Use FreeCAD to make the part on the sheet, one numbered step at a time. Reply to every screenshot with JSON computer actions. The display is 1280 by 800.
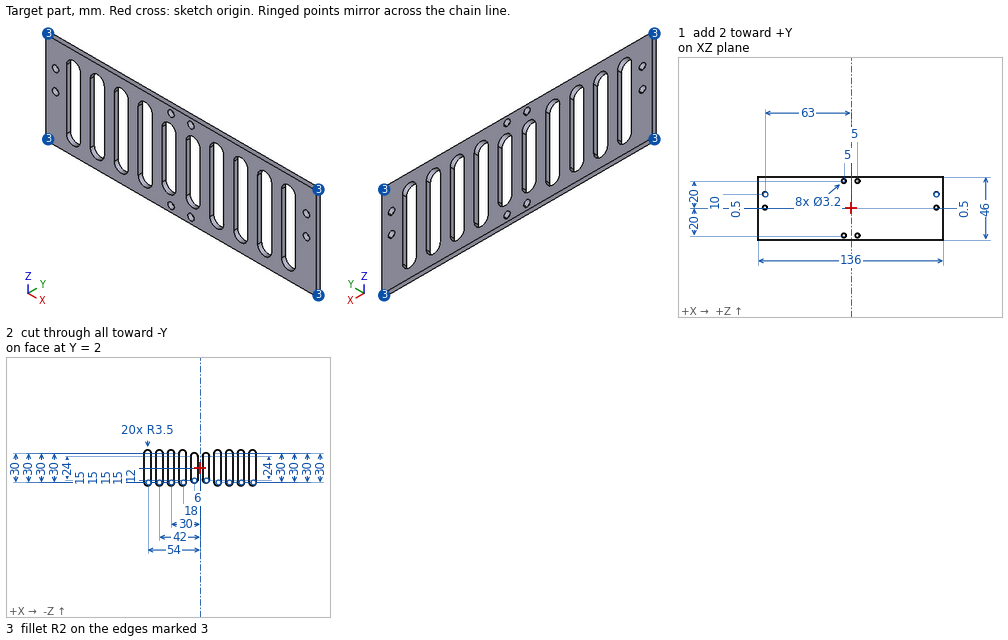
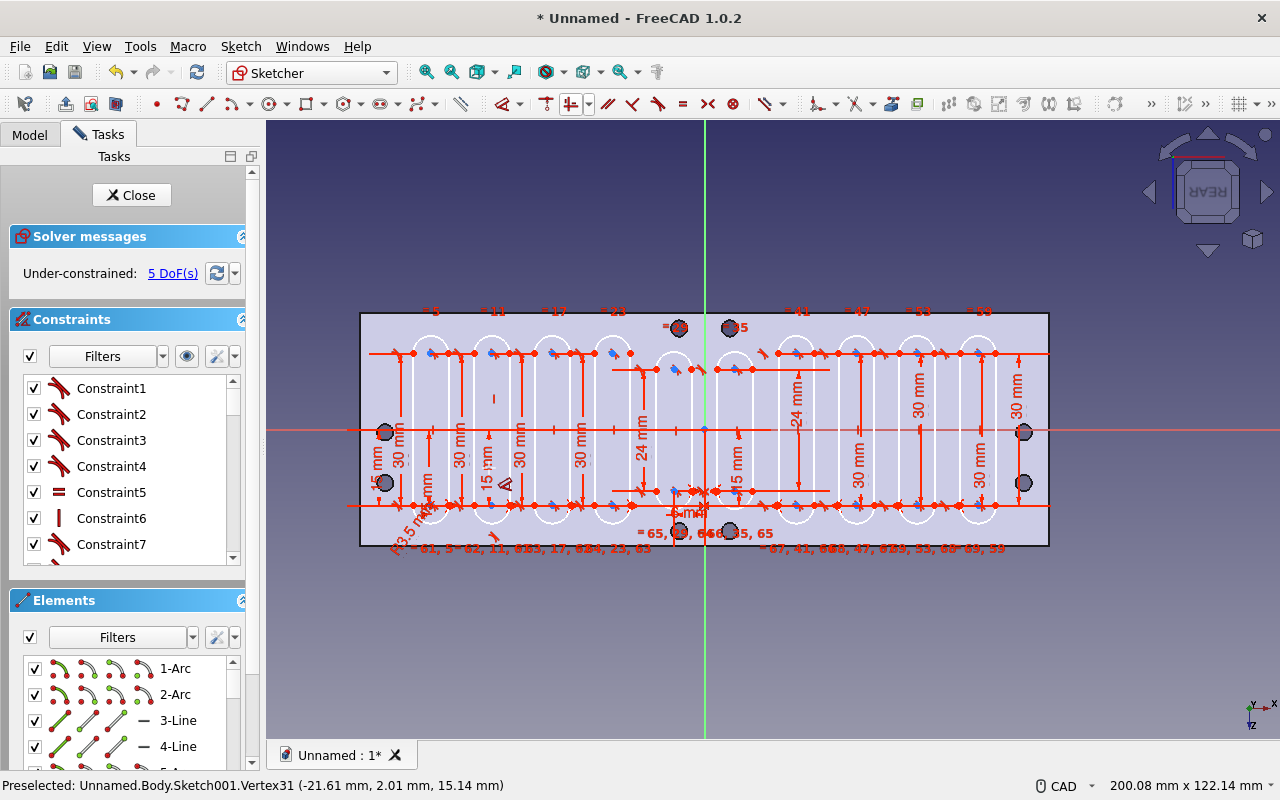
{"action": "left_click", "coordinate": [656, 491]}
{"action": "left_click", "coordinate": [739, 446]}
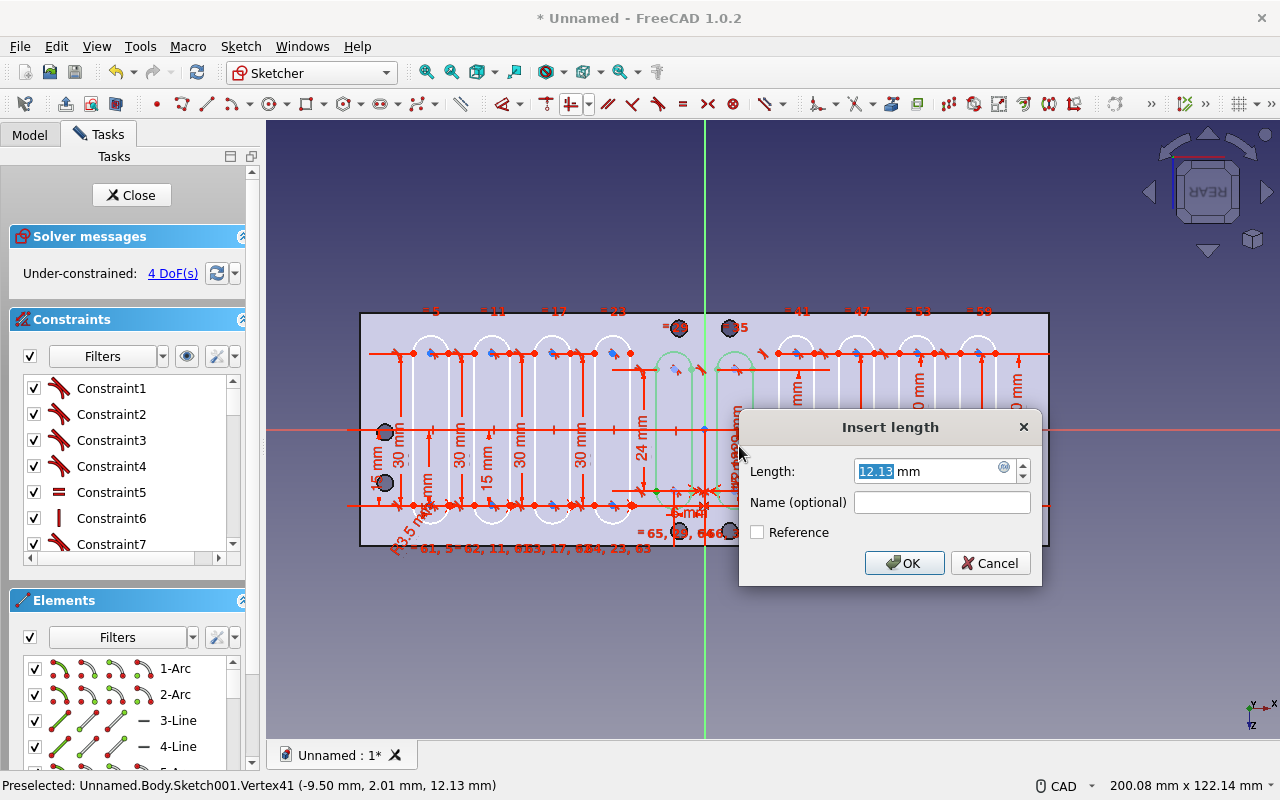
{"action": "type", "text": "12"}
{"action": "key", "text": "Return"}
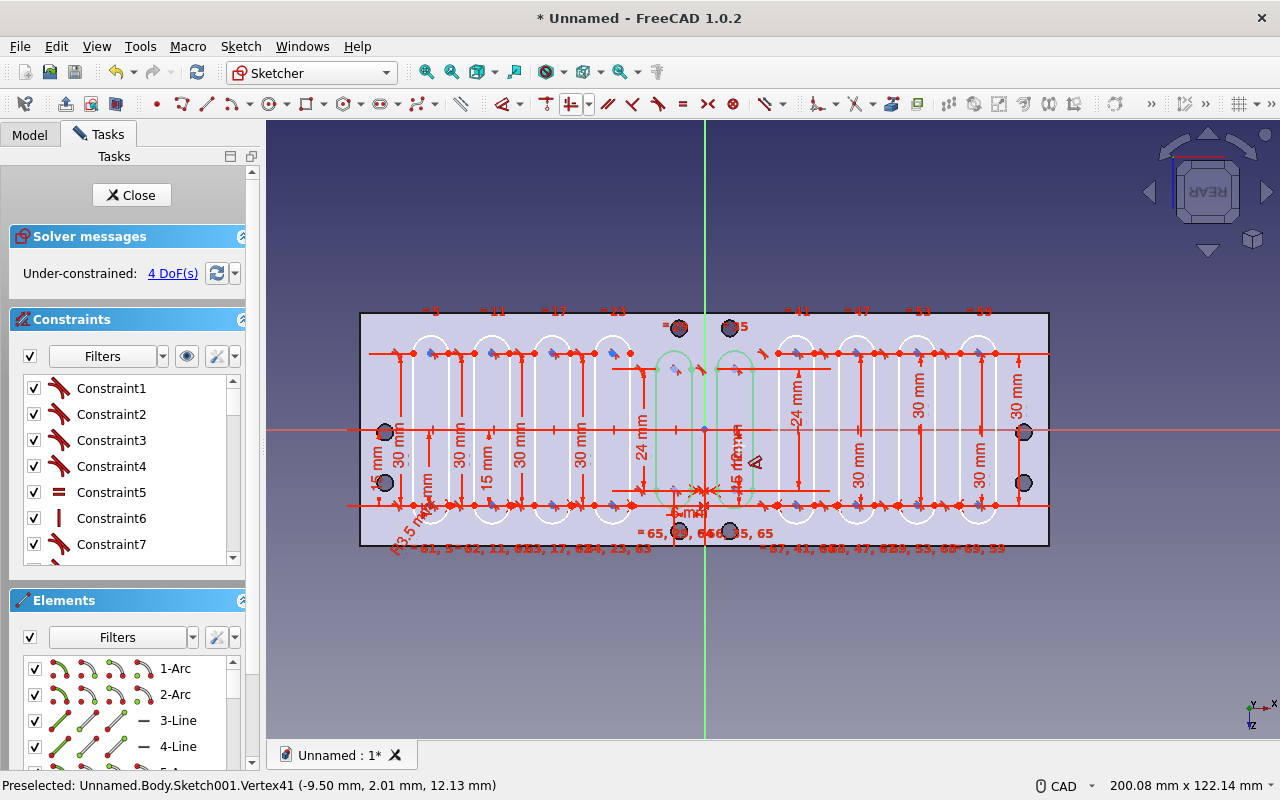
{"action": "left_click", "coordinate": [431, 506]}
{"action": "left_click", "coordinate": [568, 540]}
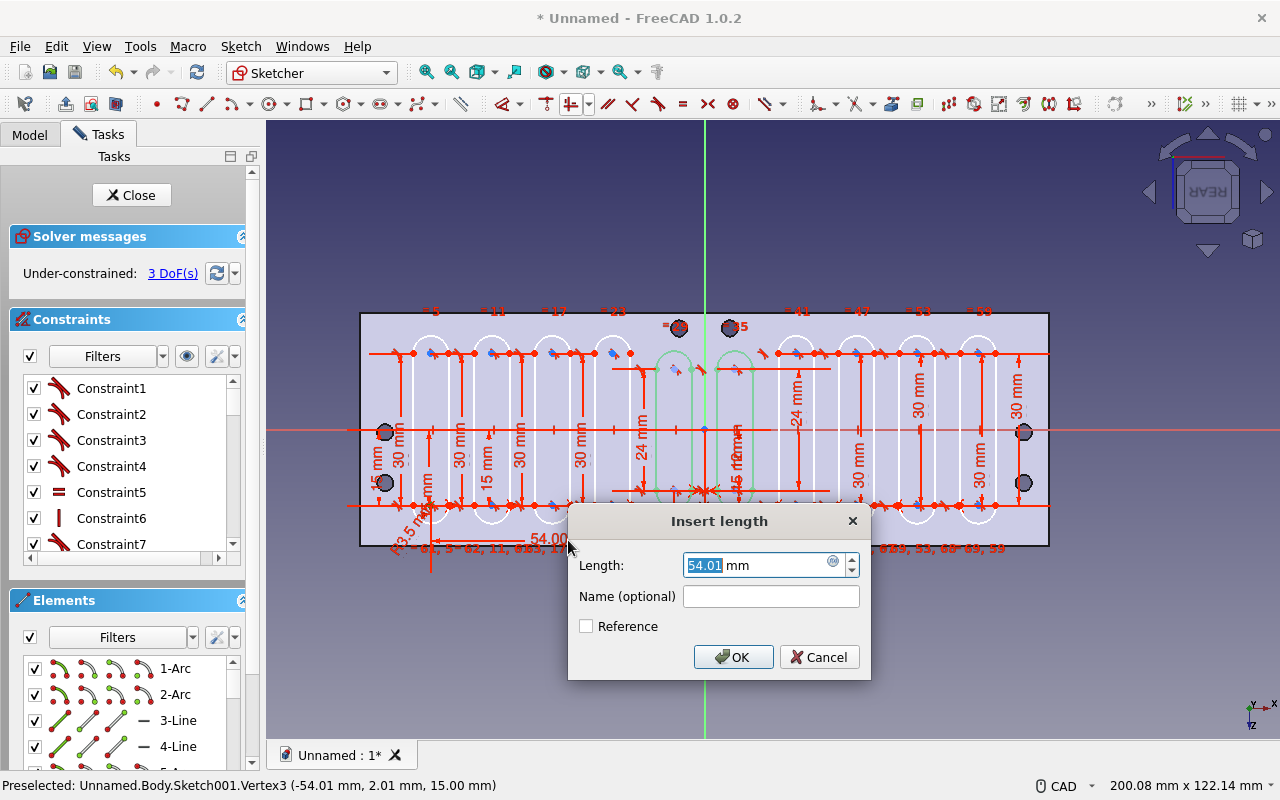
{"action": "type", "text": "54"}
{"action": "key", "text": "Return"}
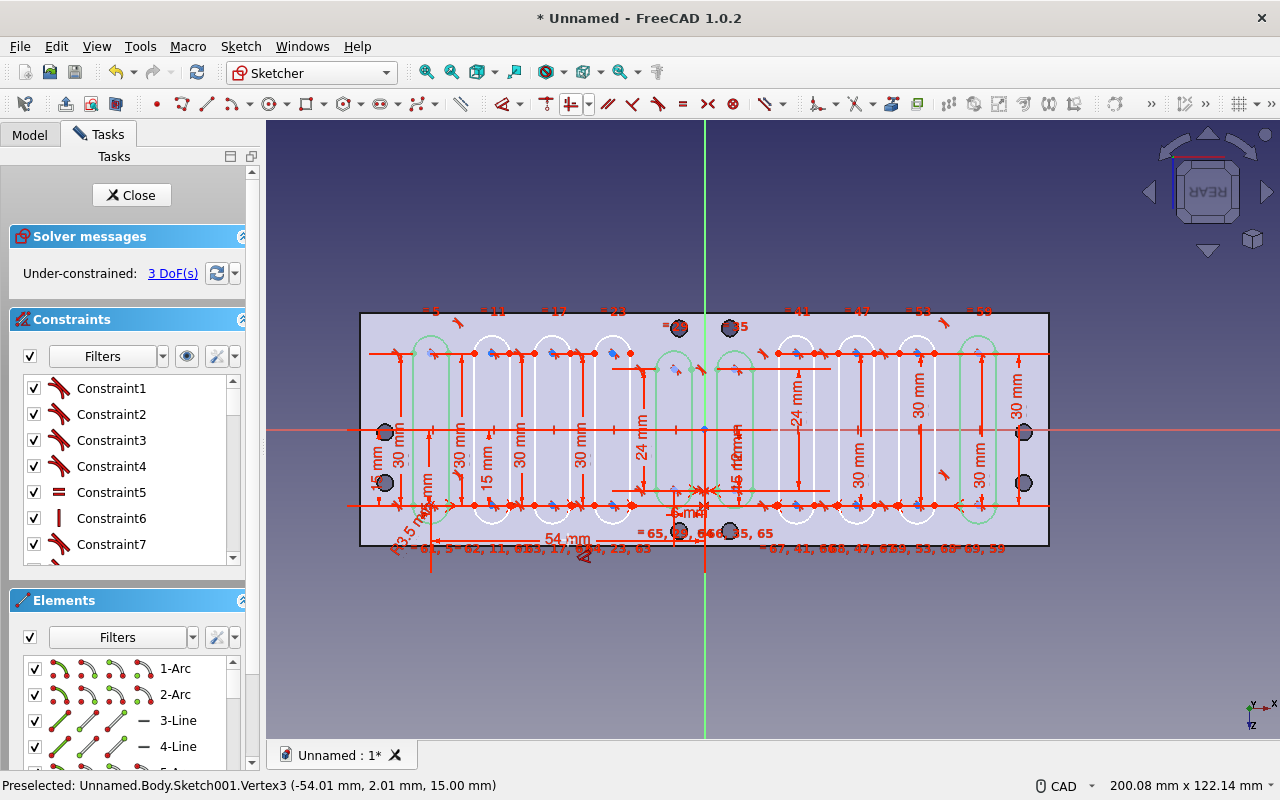
{"action": "left_click", "coordinate": [492, 506]}
{"action": "left_click", "coordinate": [647, 540]}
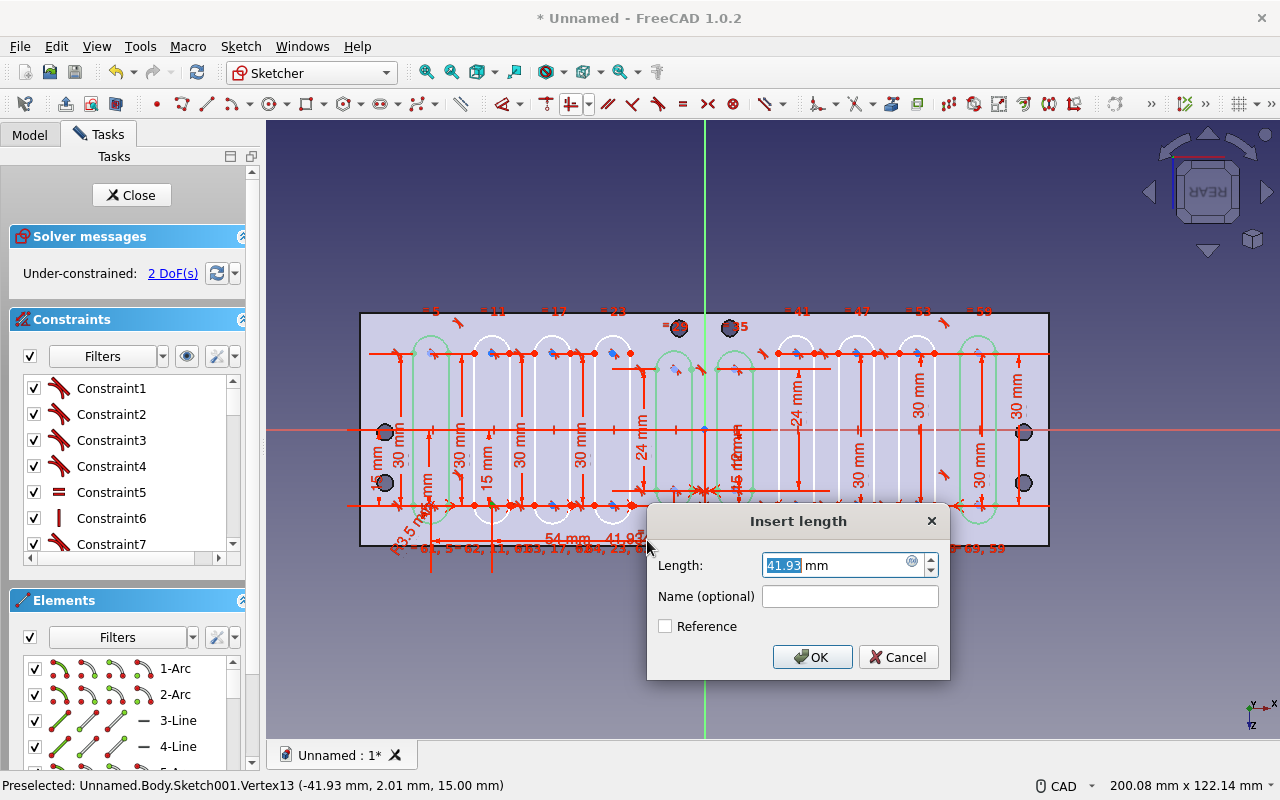
{"action": "type", "text": "42"}
{"action": "key", "text": "Return"}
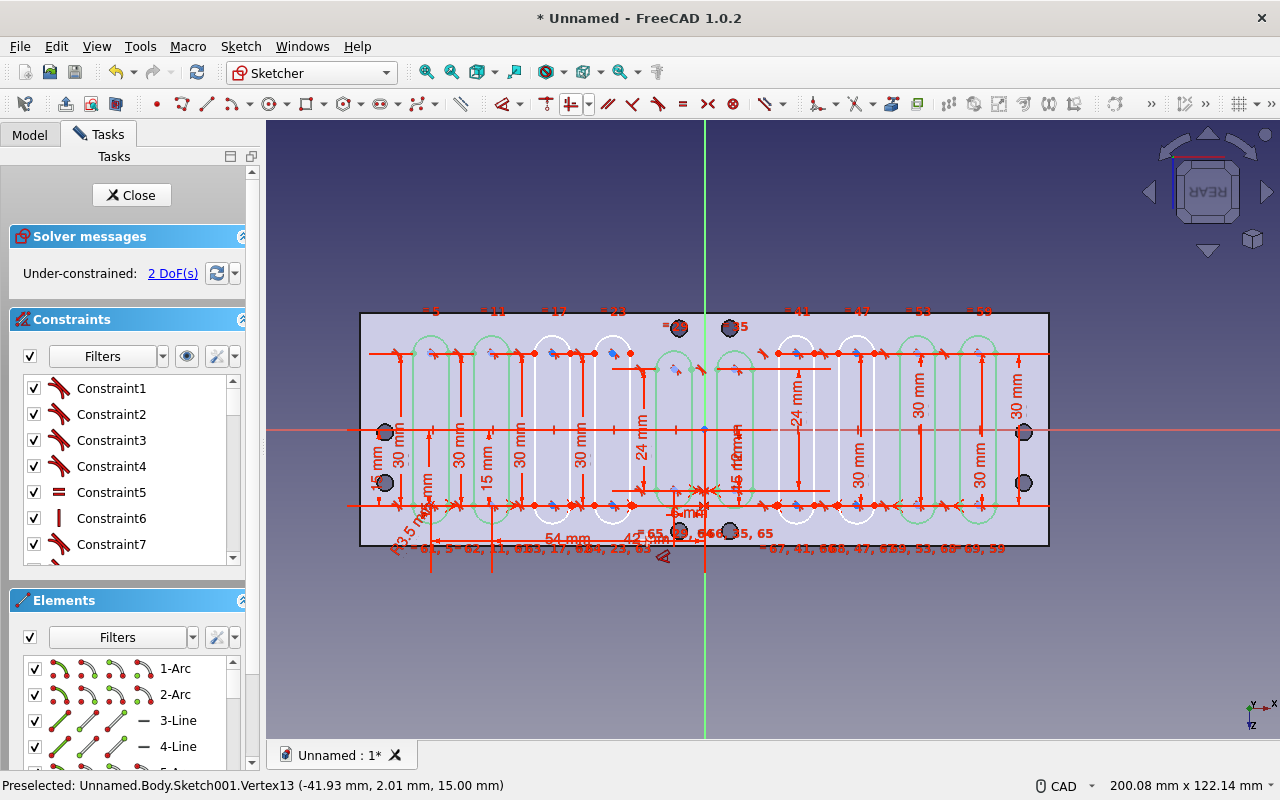
{"action": "left_click", "coordinate": [552, 506]}
{"action": "left_click", "coordinate": [628, 564]}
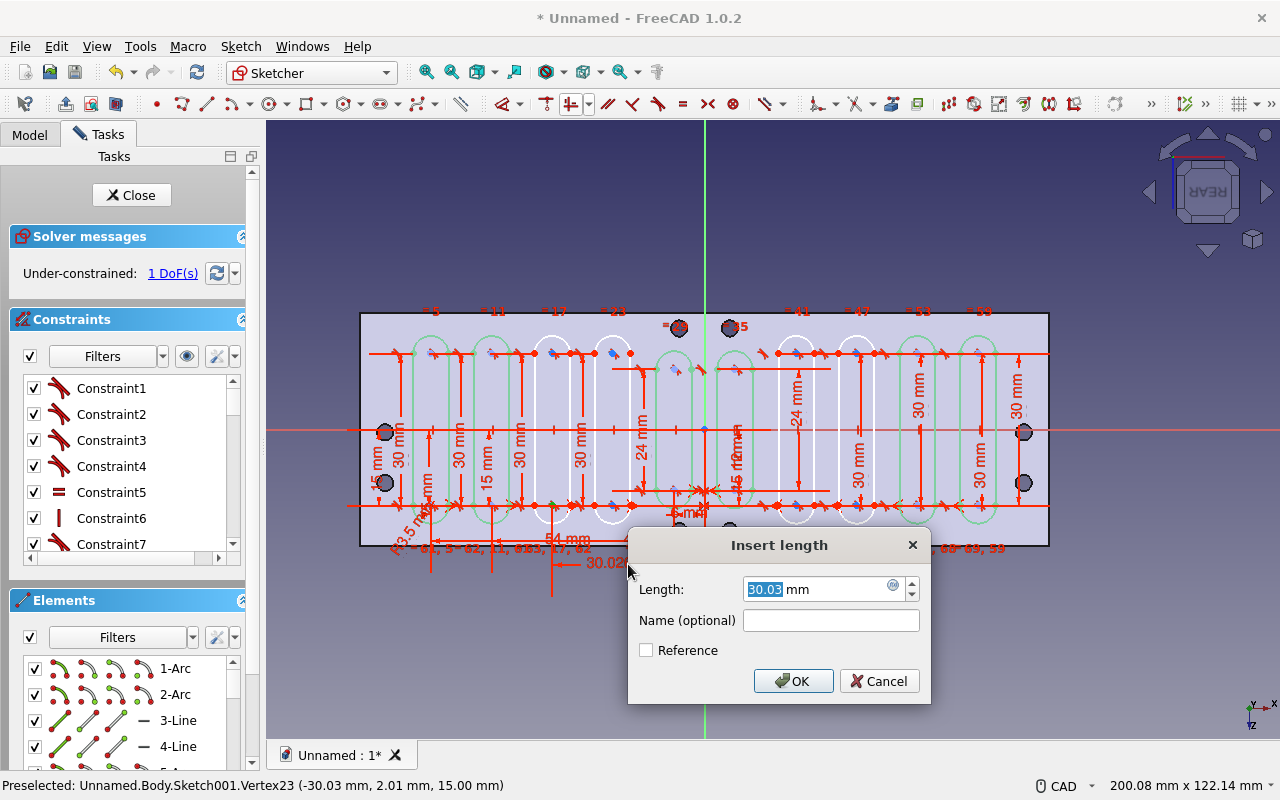
{"action": "type", "text": "30"}
{"action": "key", "text": "Return"}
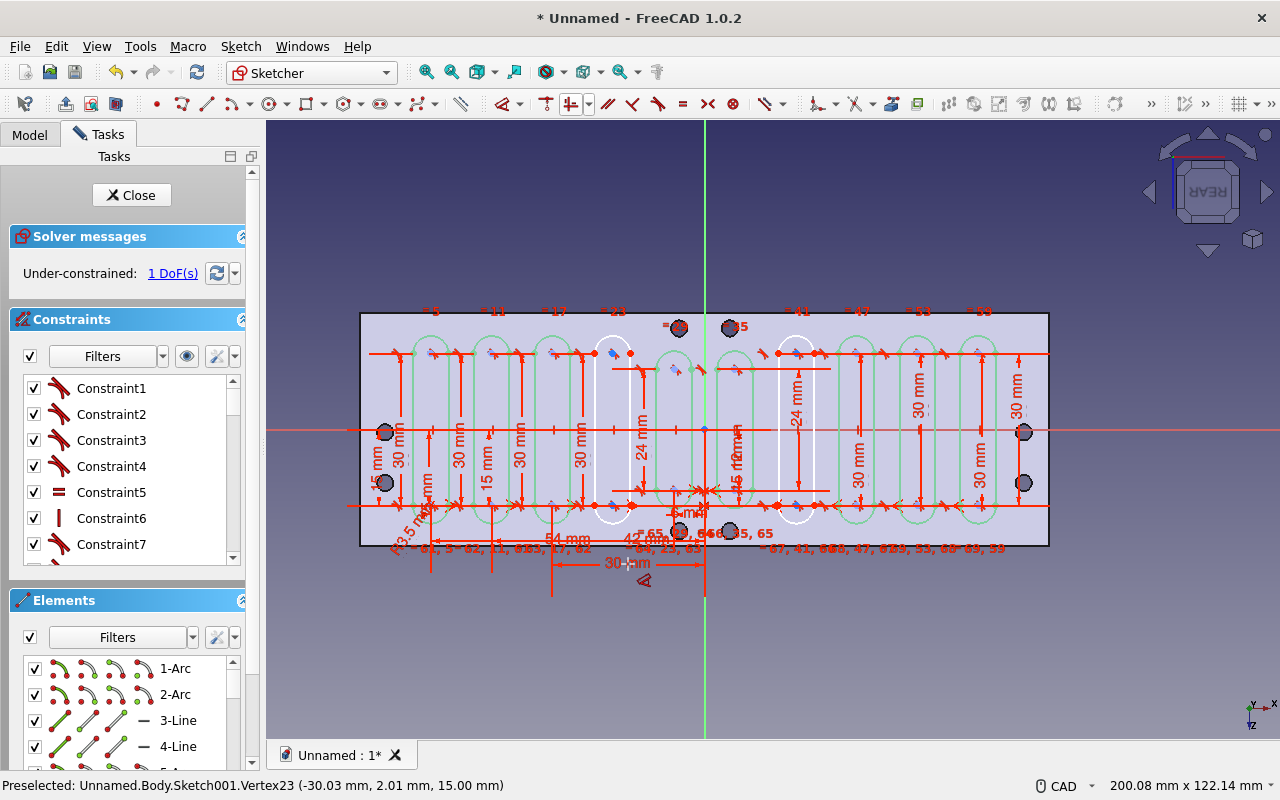
{"action": "left_click", "coordinate": [613, 506]}
{"action": "left_click", "coordinate": [659, 588]}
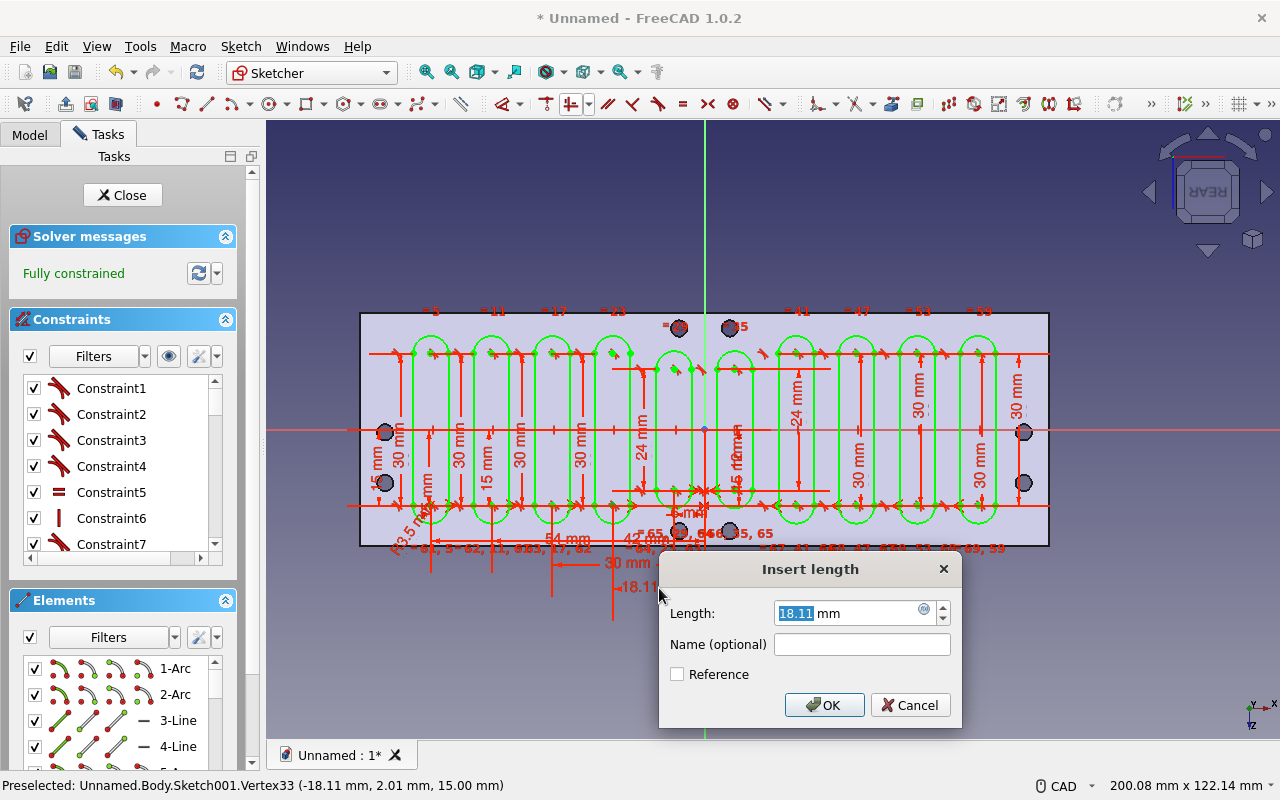
{"action": "type", "text": "18"}
{"action": "key", "text": "Return"}
{"action": "key", "text": "Escape"}